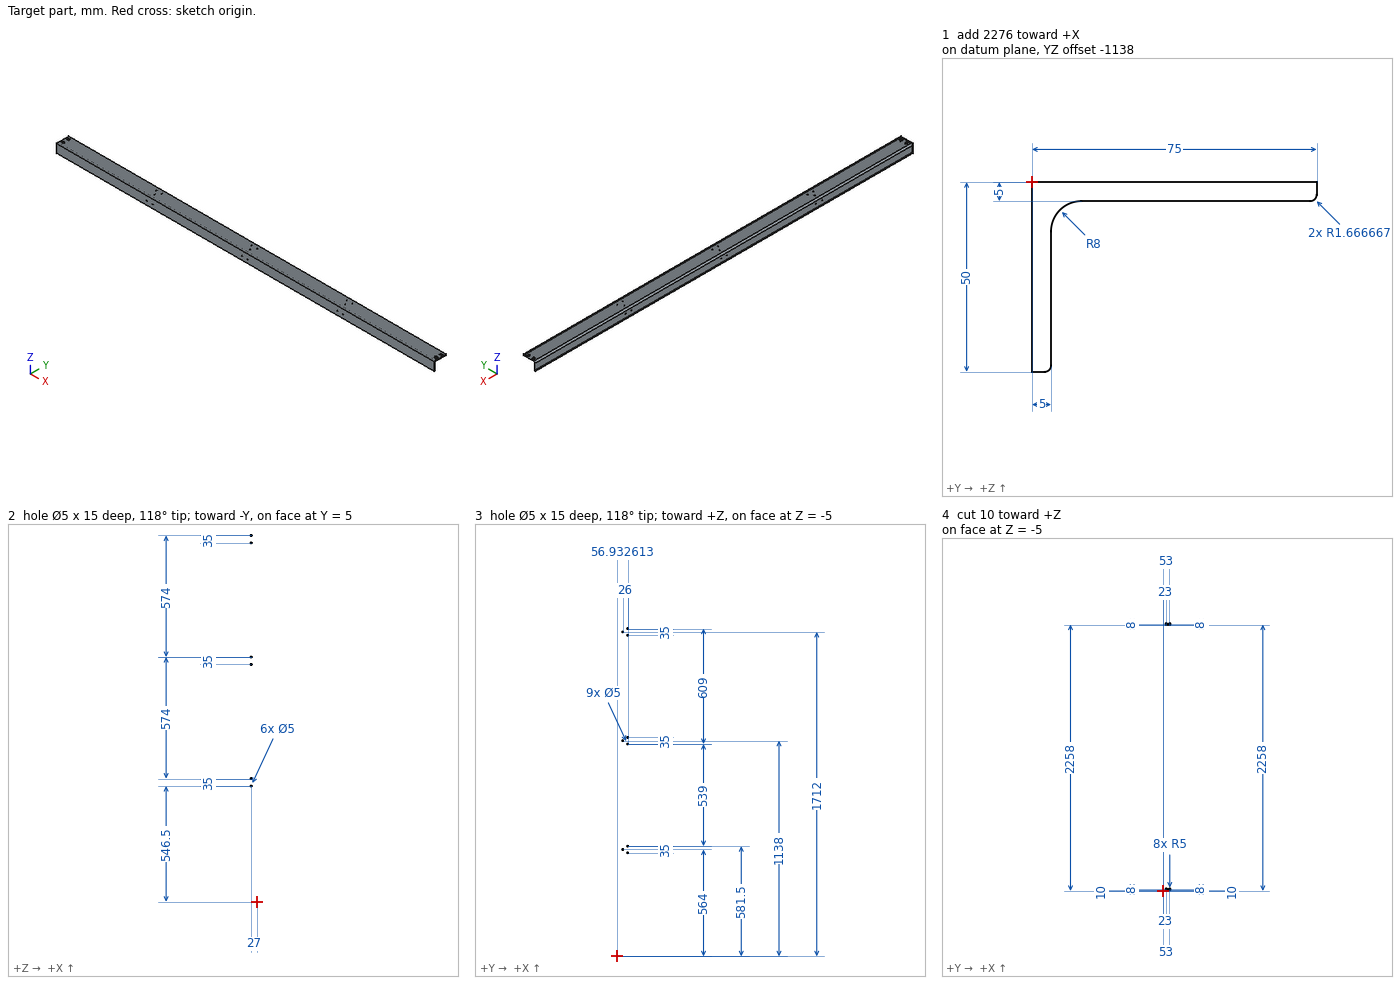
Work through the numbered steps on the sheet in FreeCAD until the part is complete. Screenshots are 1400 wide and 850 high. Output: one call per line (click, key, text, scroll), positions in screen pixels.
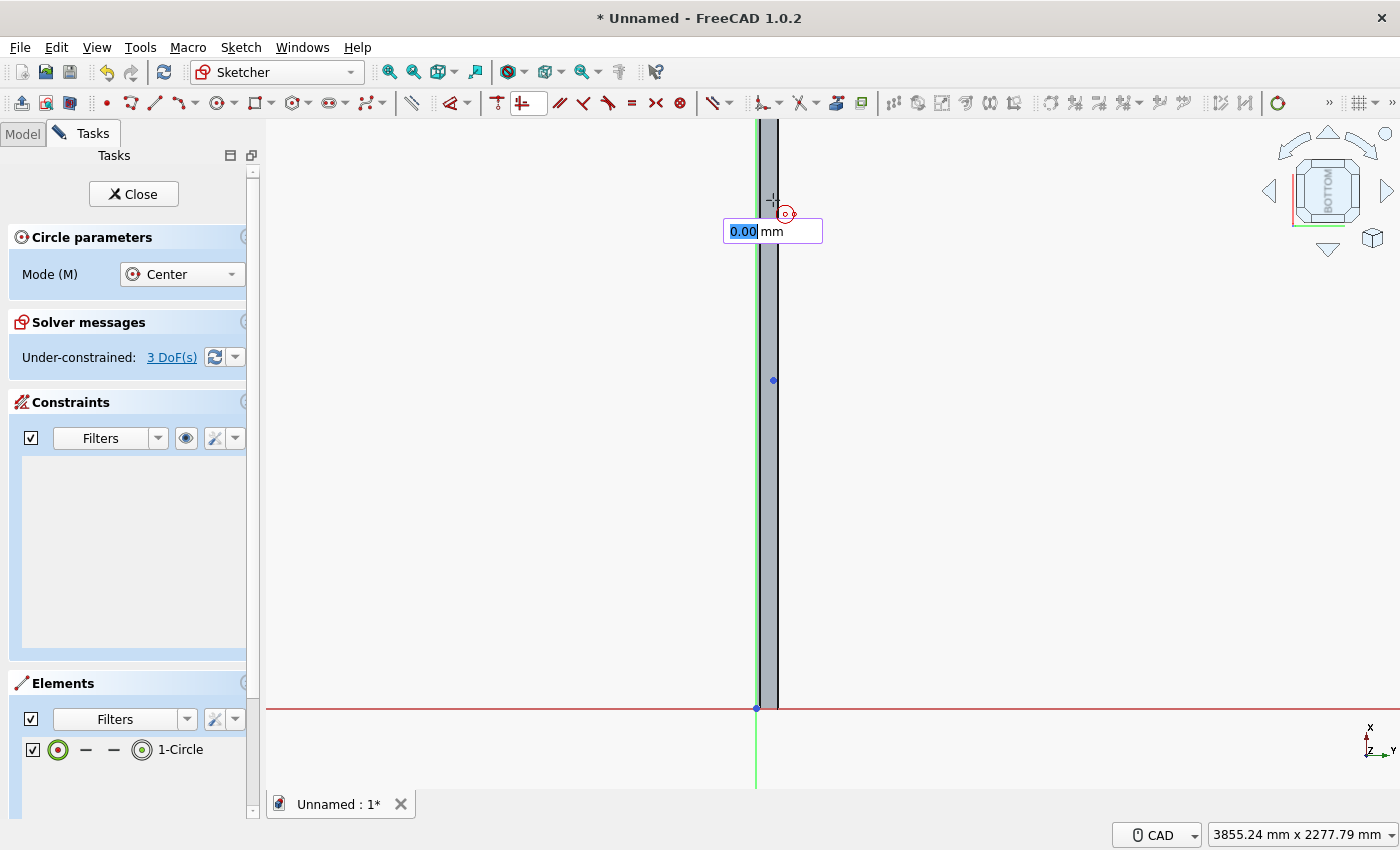
scroll(773, 199, up, 16)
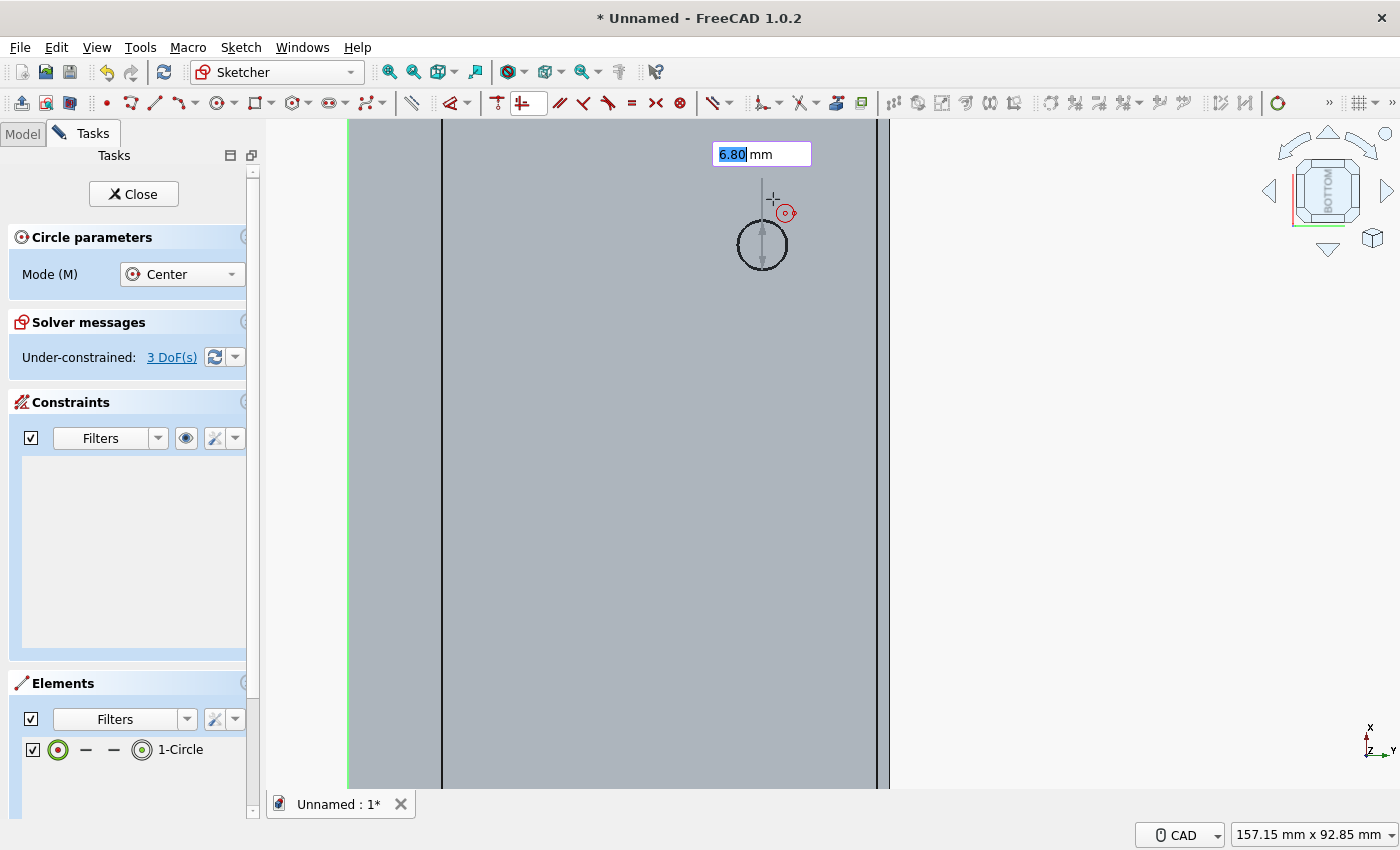
click(772, 205)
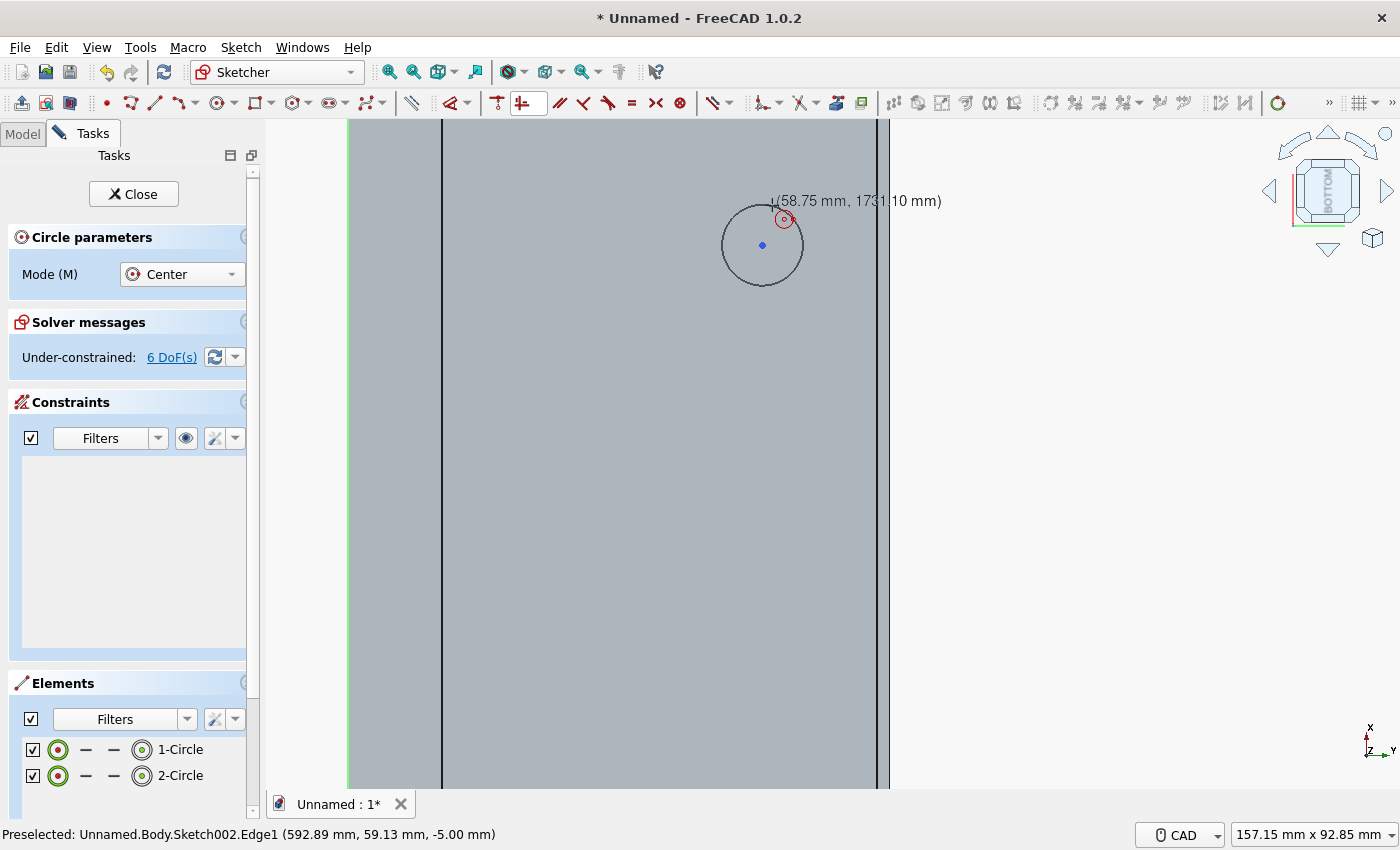
scroll(759, 470, up, 2)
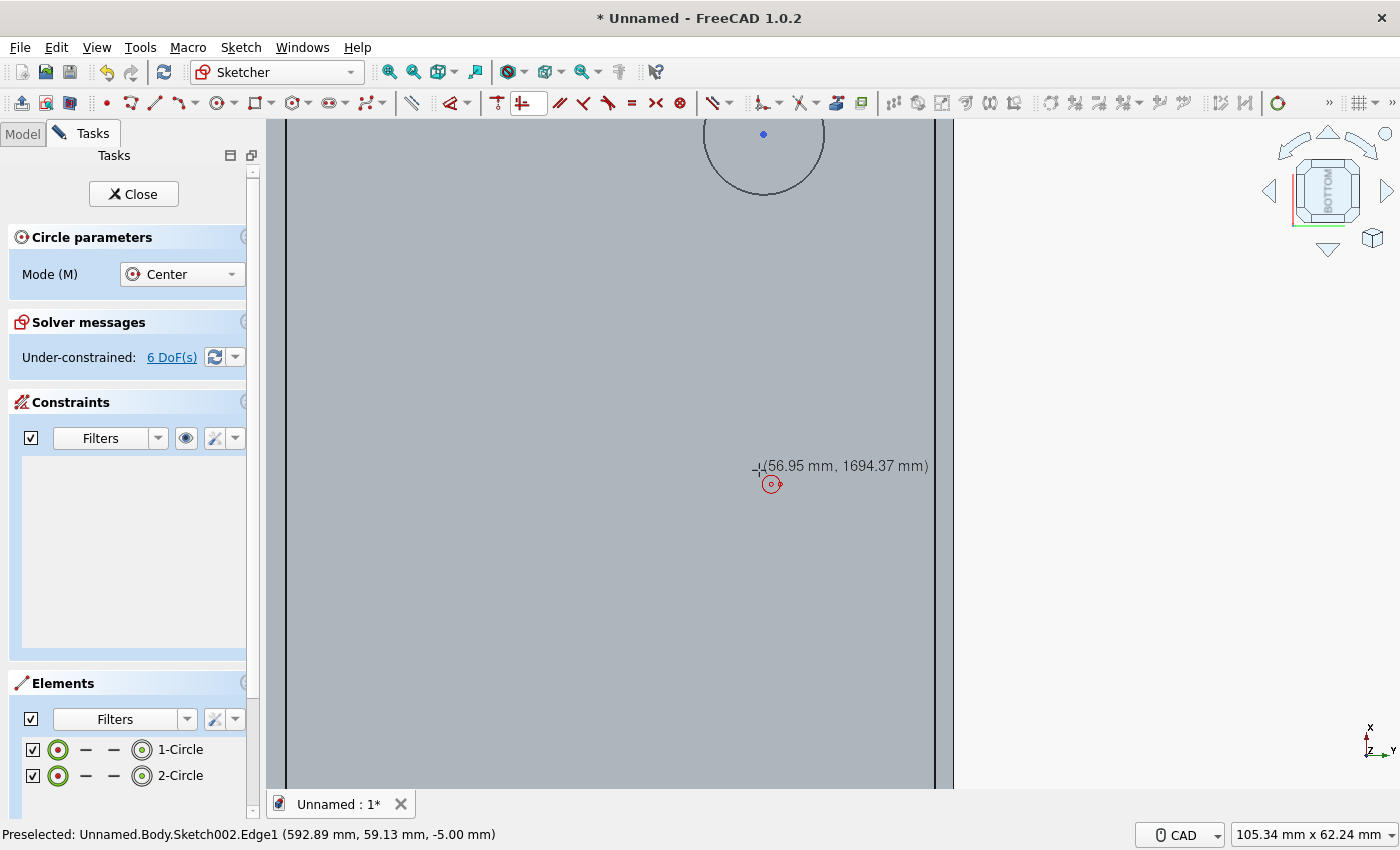
scroll(773, 203, down, 18)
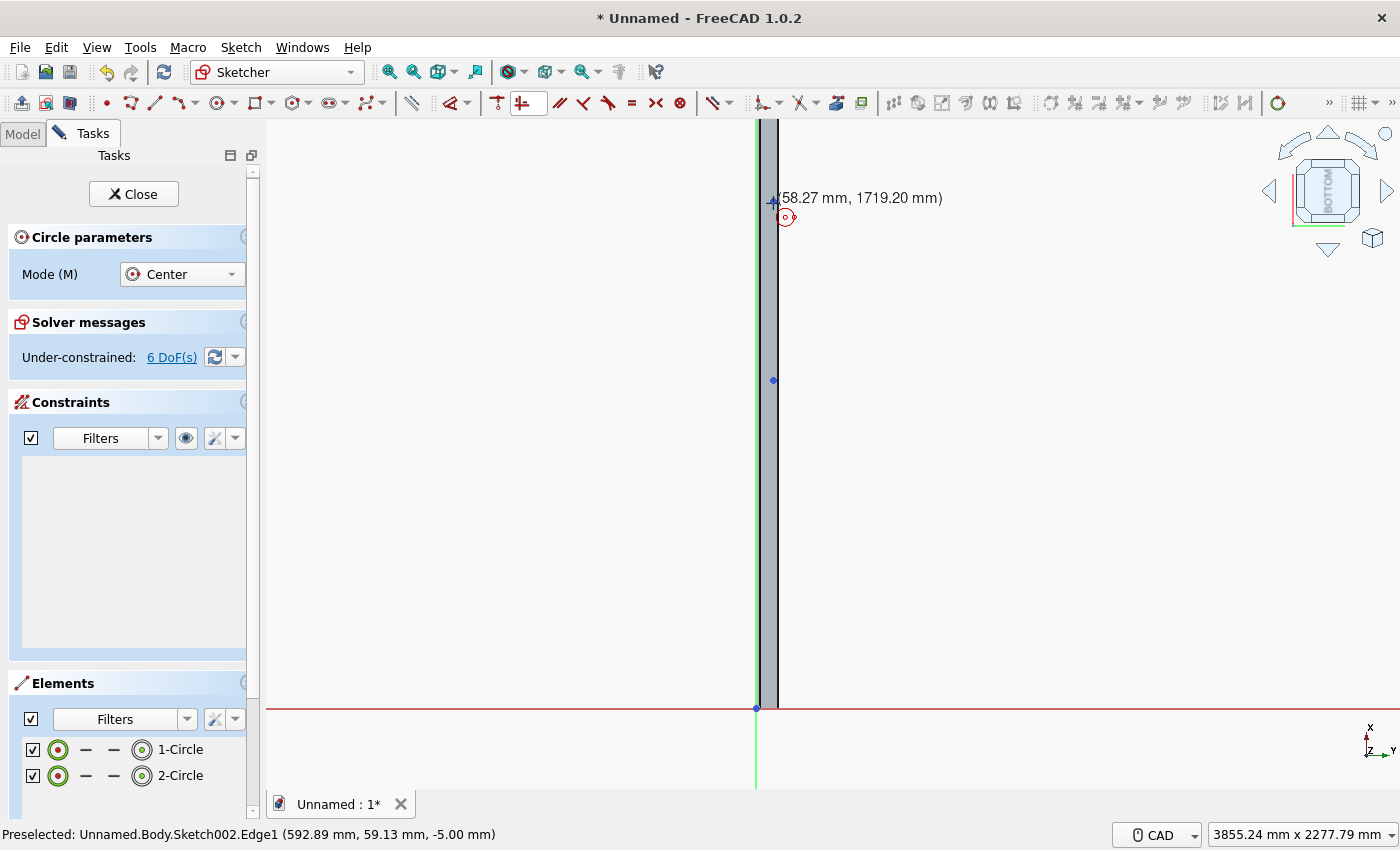
scroll(773, 210, up, 3)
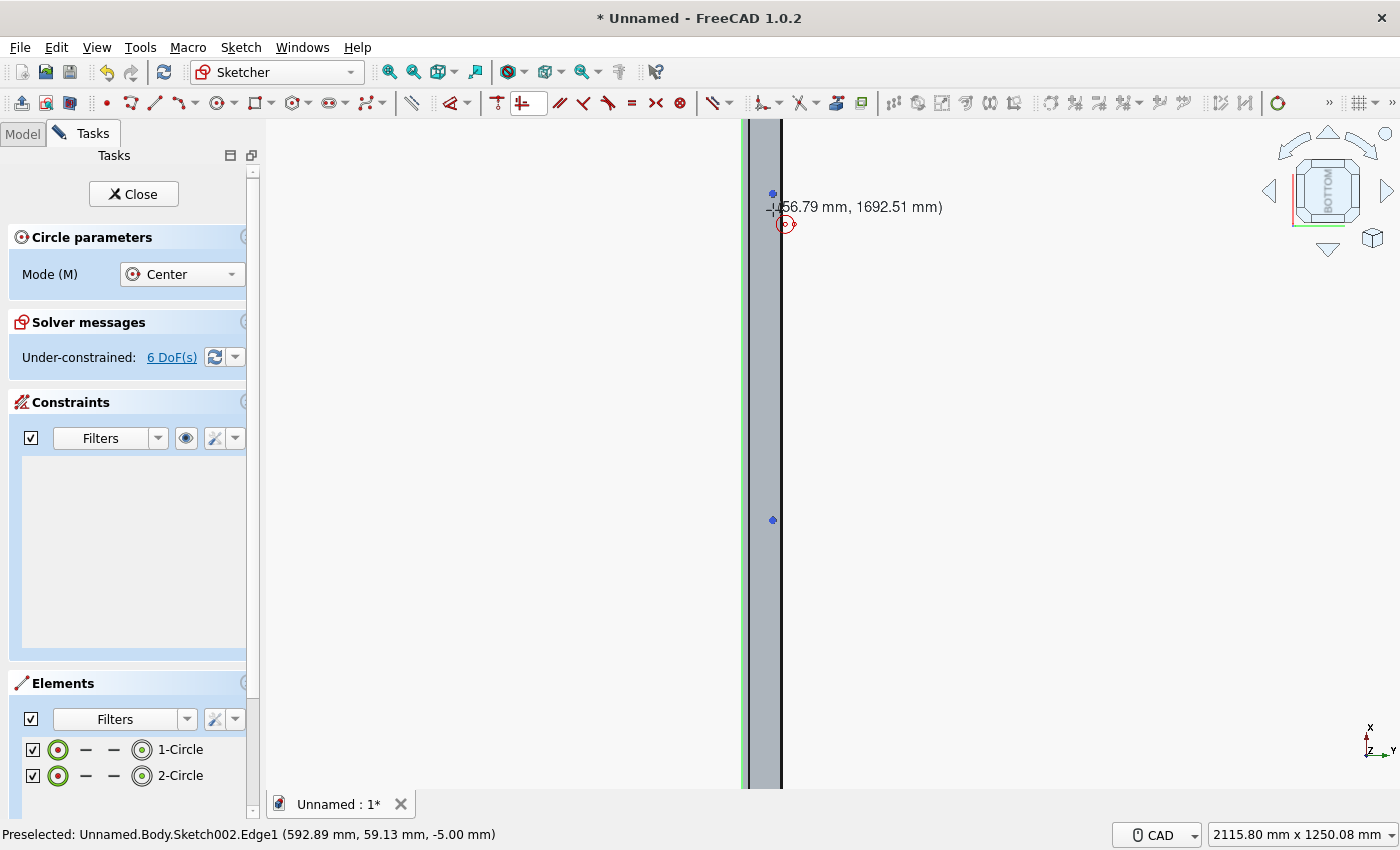
click(773, 211)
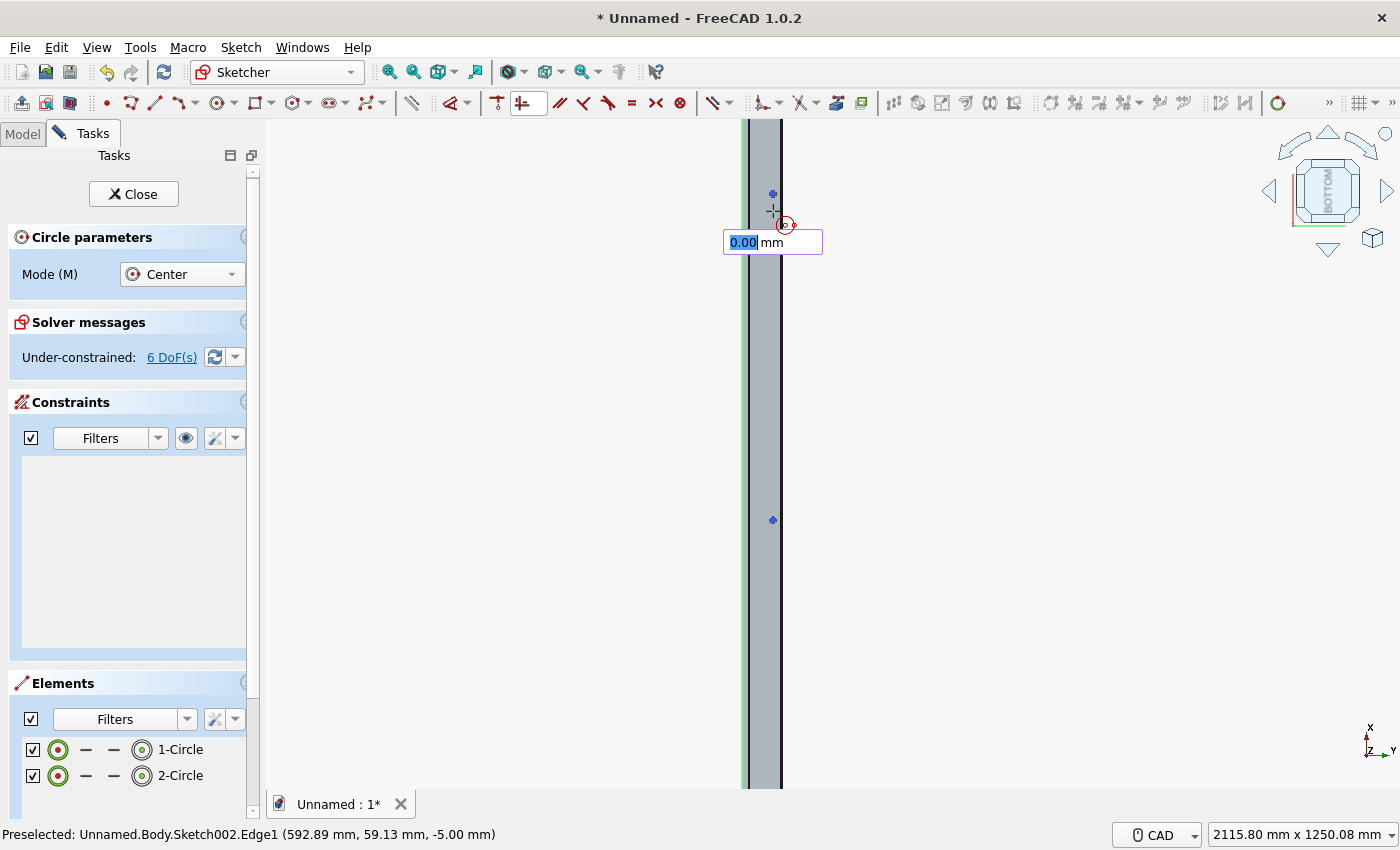
scroll(774, 210, up, 13)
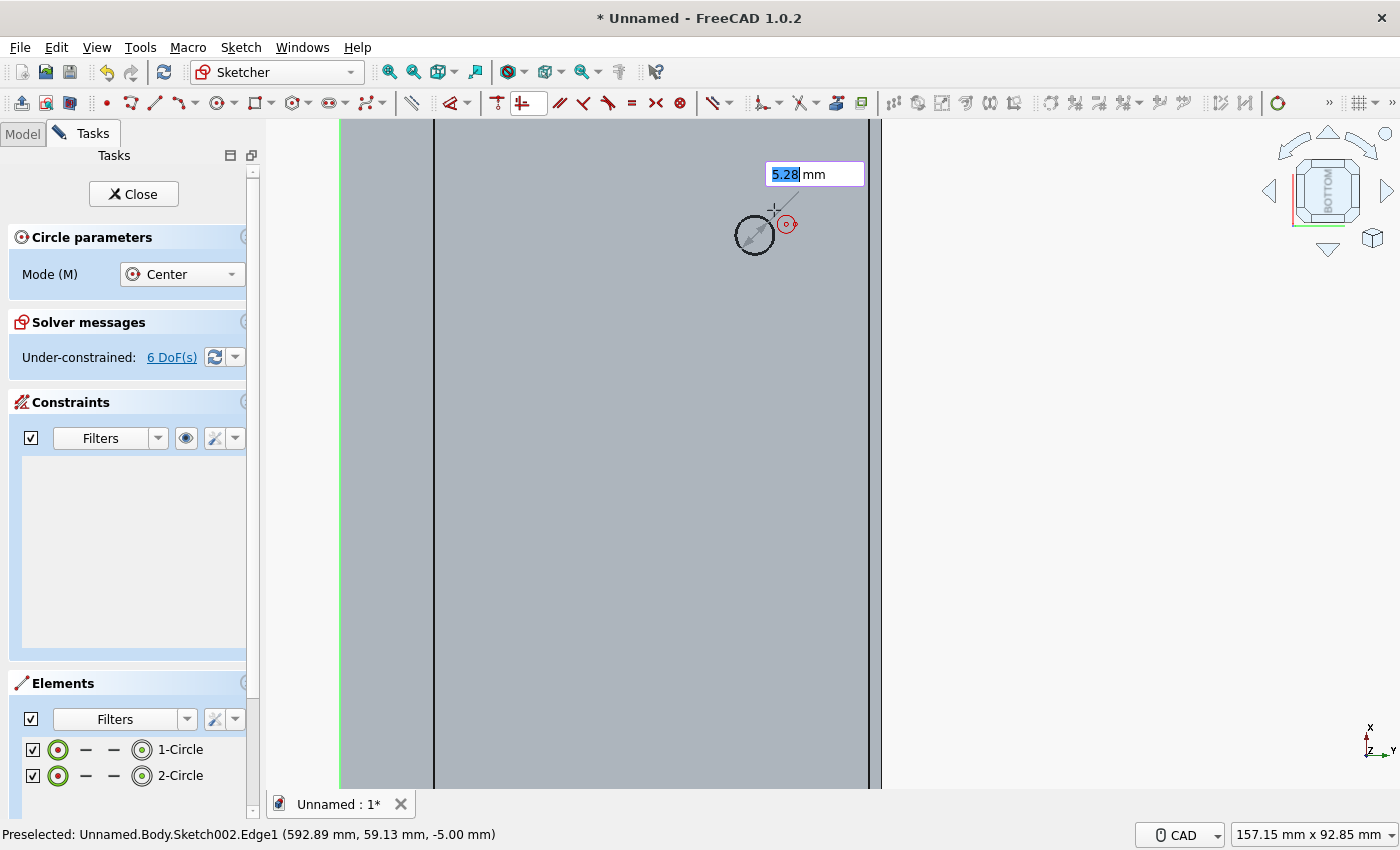
click(764, 204)